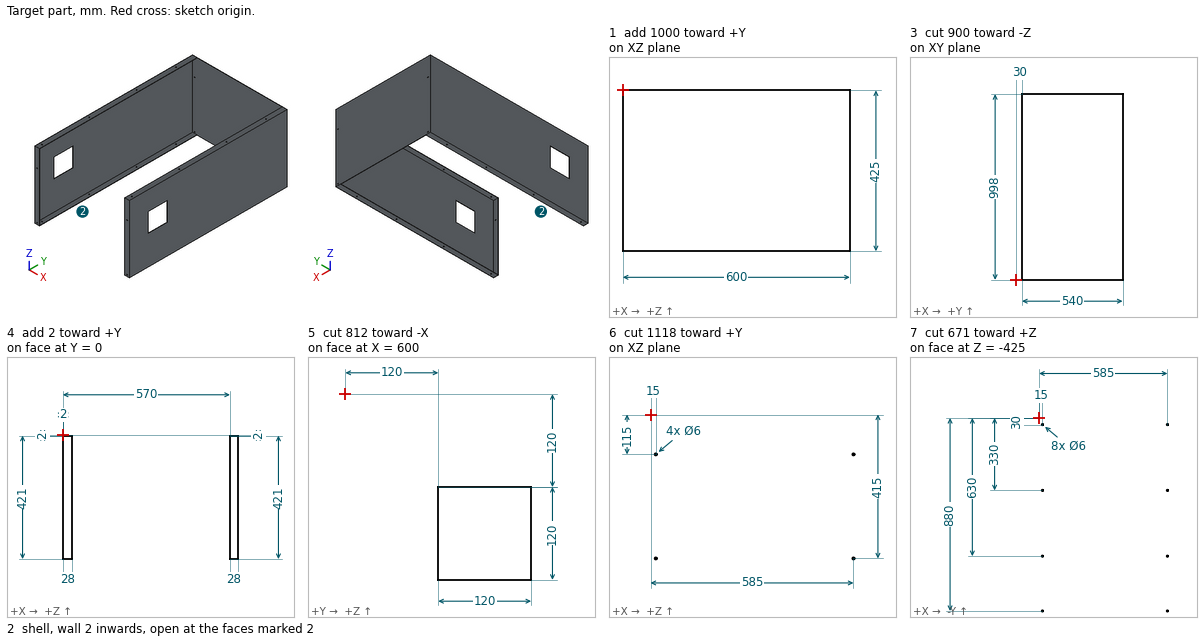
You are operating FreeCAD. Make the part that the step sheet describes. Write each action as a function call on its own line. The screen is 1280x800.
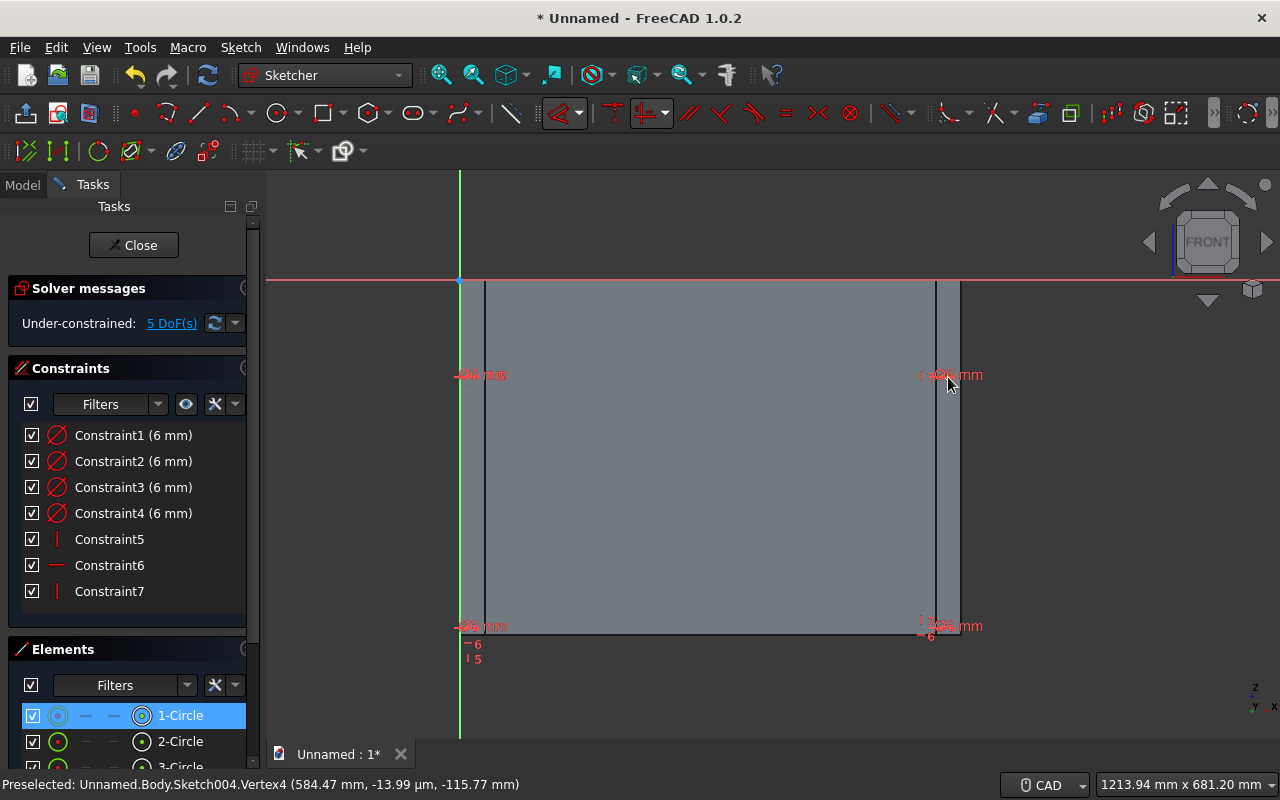
key(h)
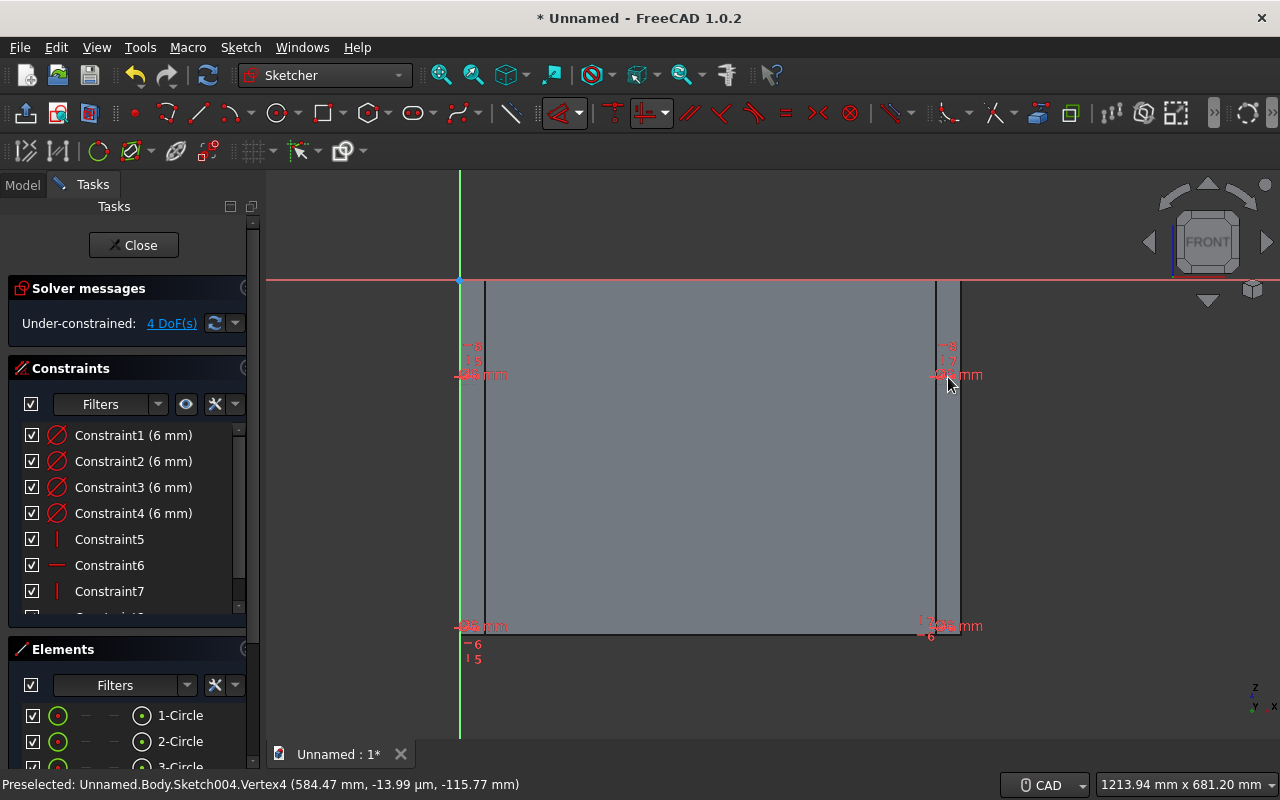
scroll(472, 377, up, 6)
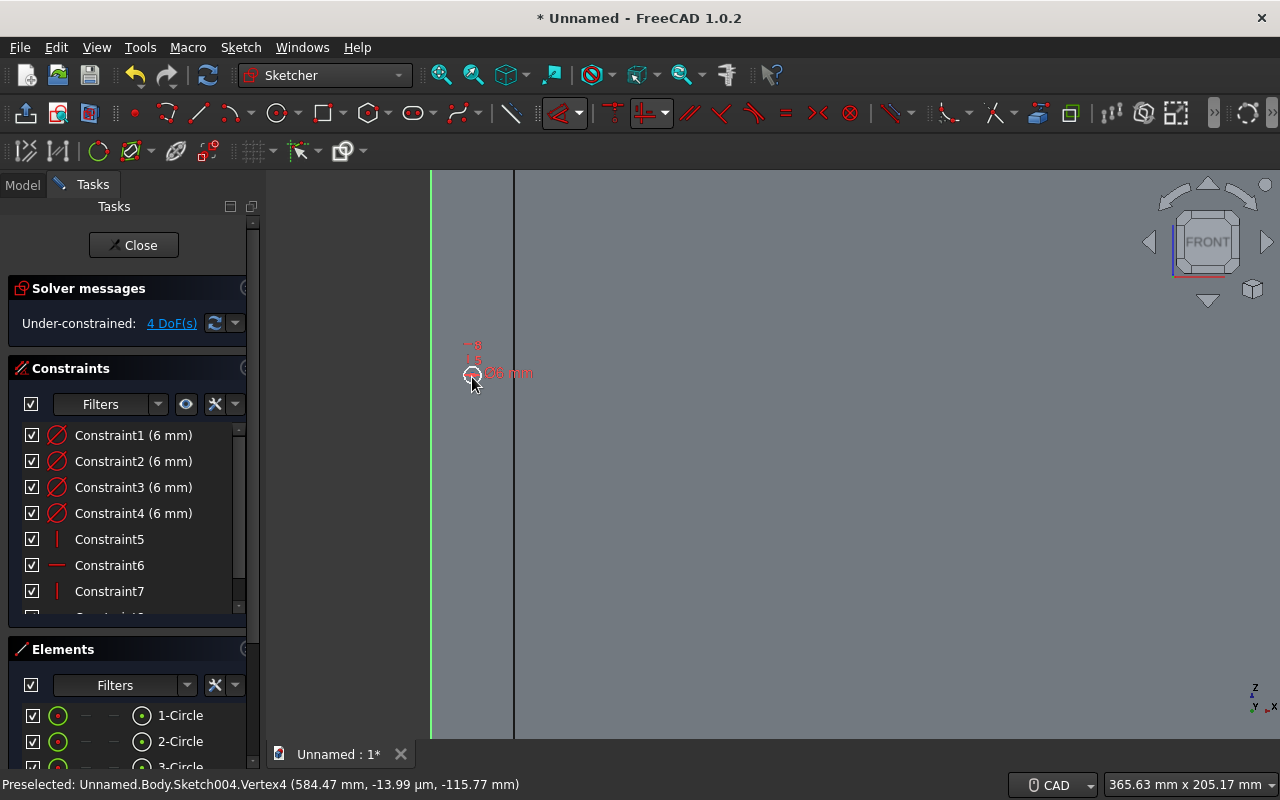
click(473, 375)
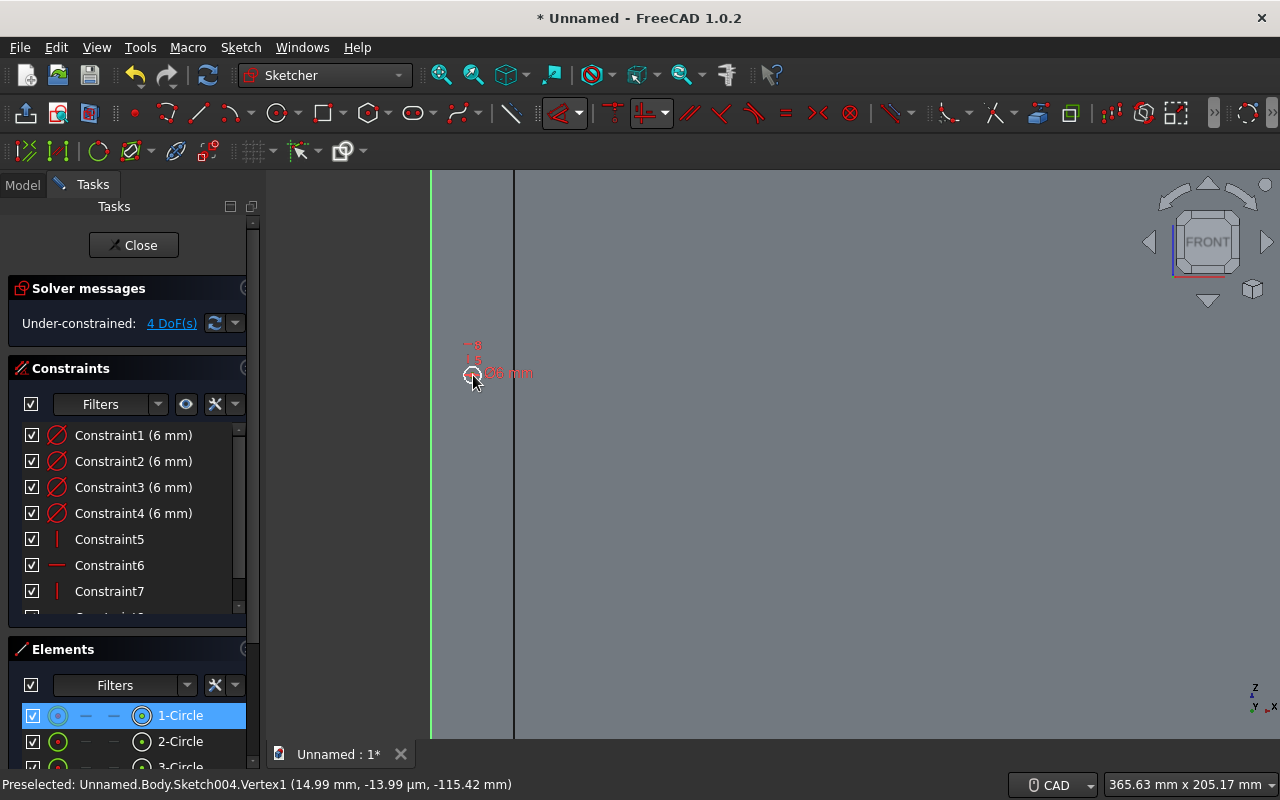
click(582, 114)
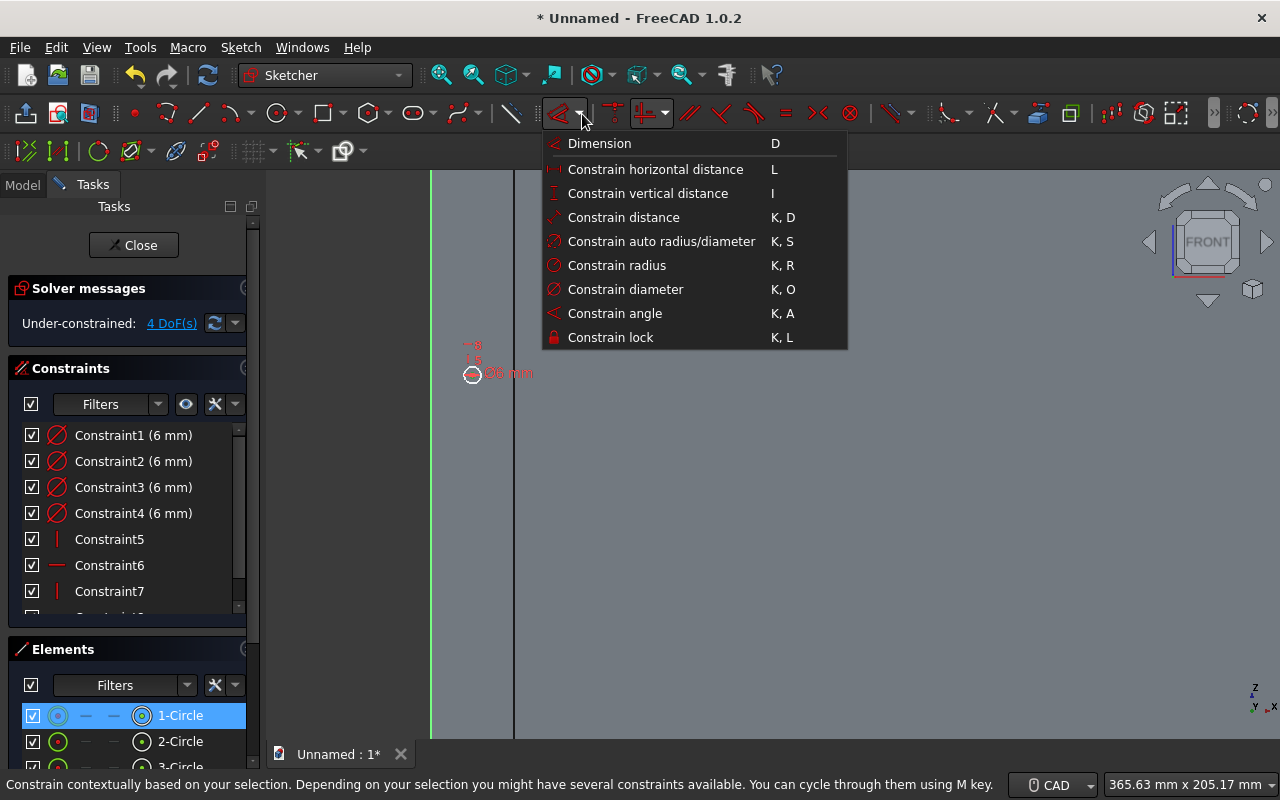
click(695, 169)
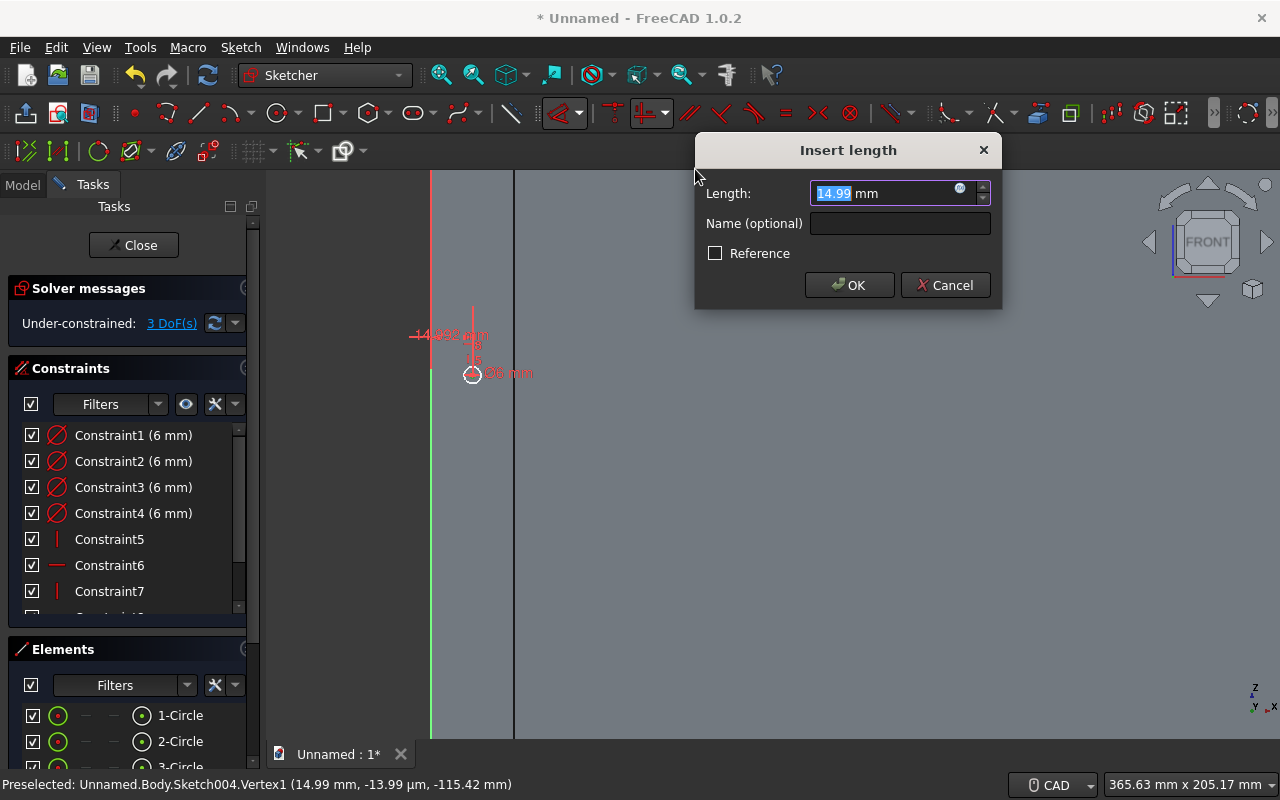
text(15)
key(Return)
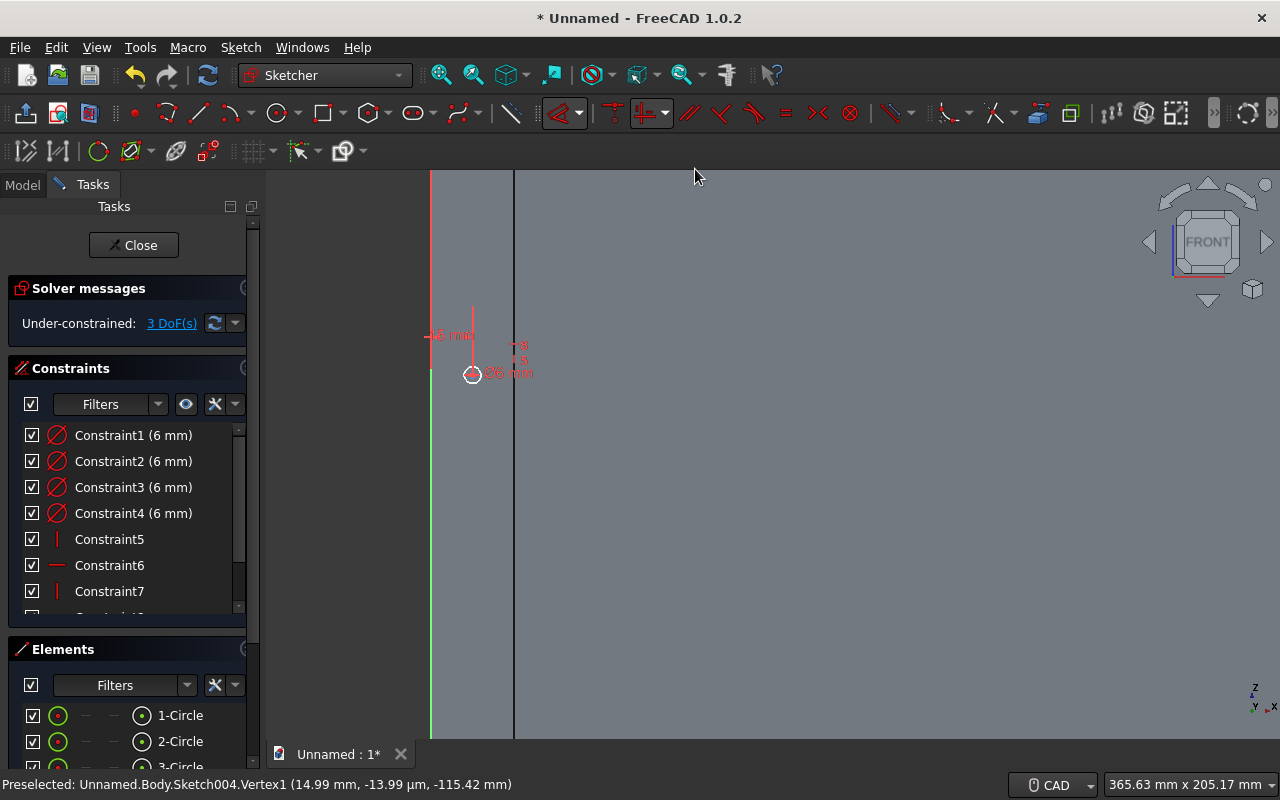
click(473, 375)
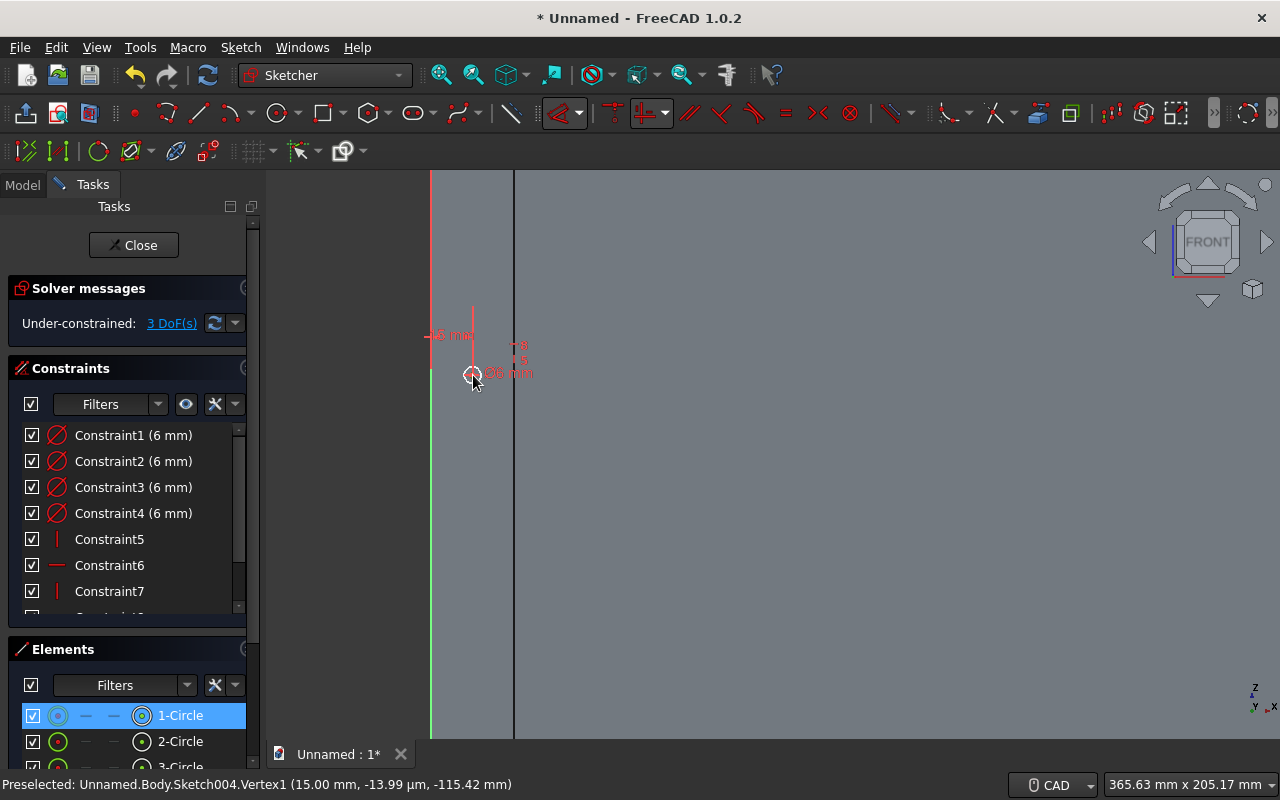
key(i)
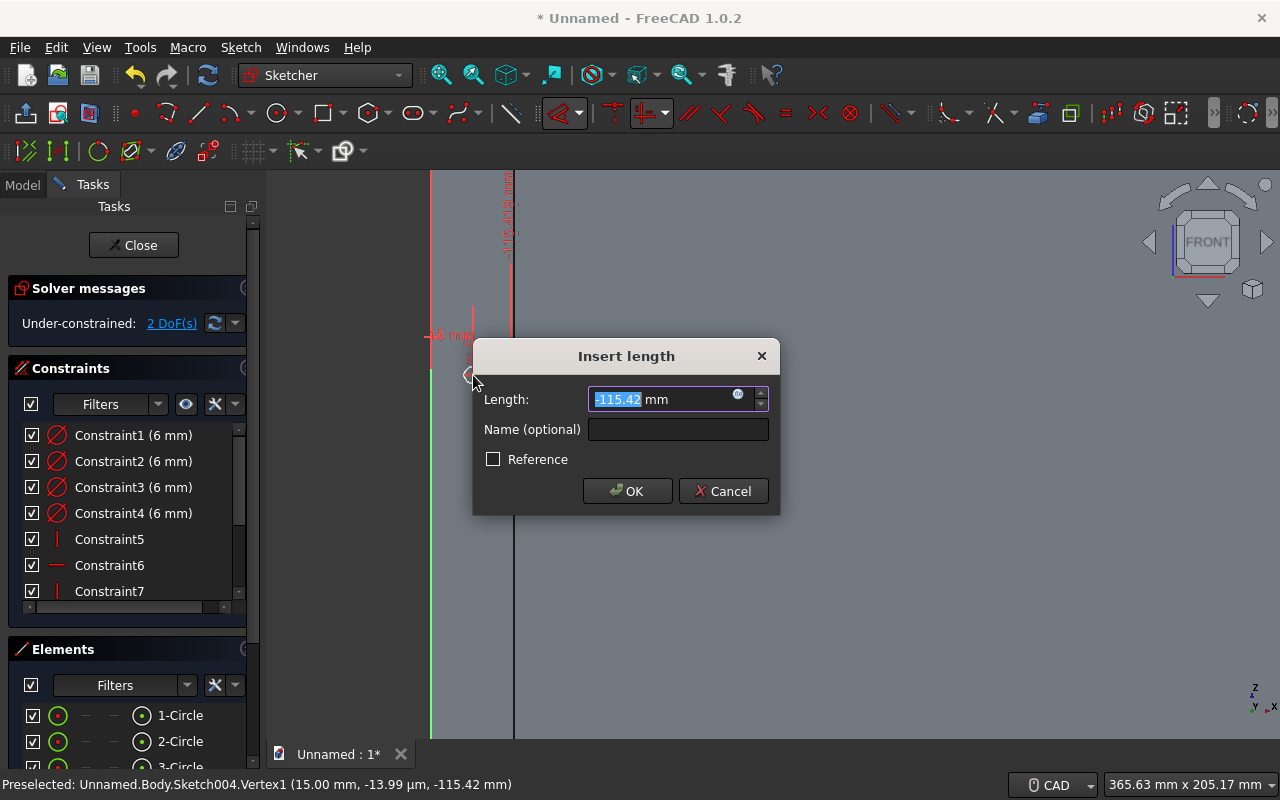
text(-115)
key(Return)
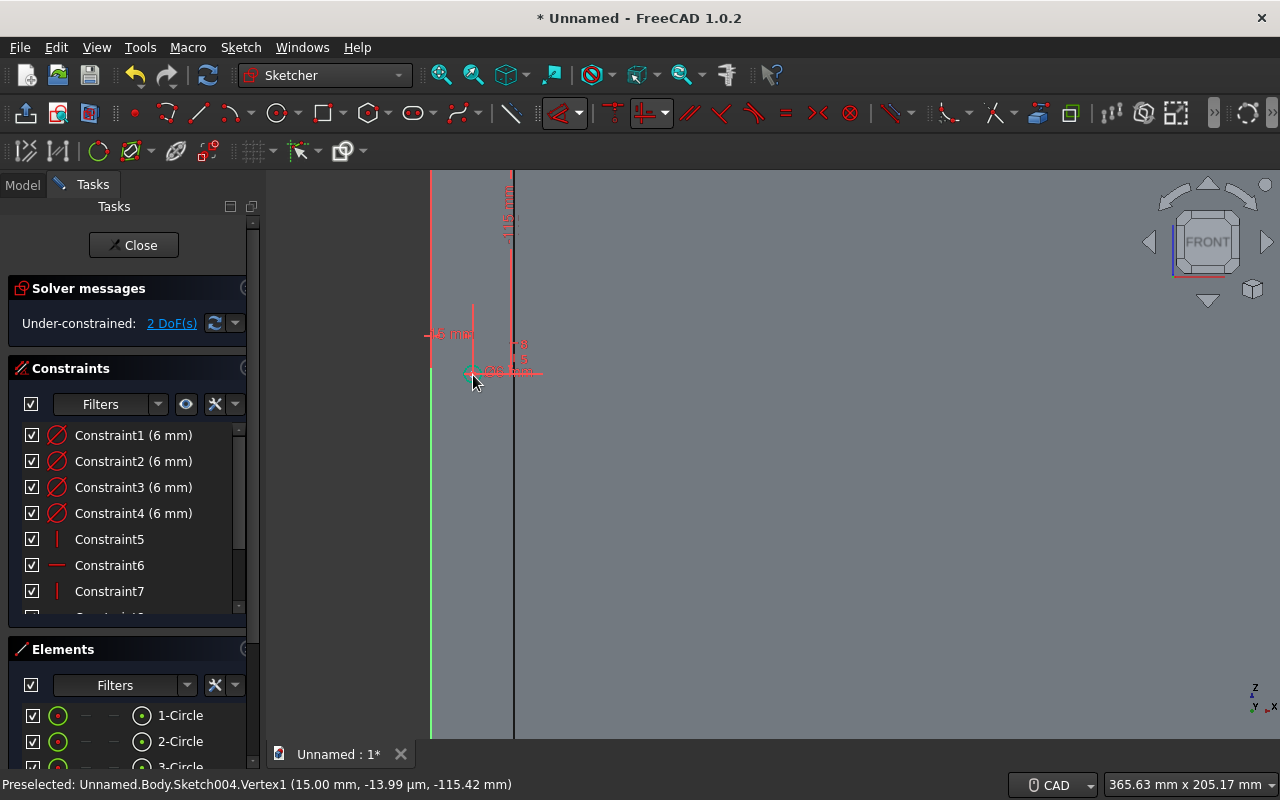
scroll(471, 377, down, 6)